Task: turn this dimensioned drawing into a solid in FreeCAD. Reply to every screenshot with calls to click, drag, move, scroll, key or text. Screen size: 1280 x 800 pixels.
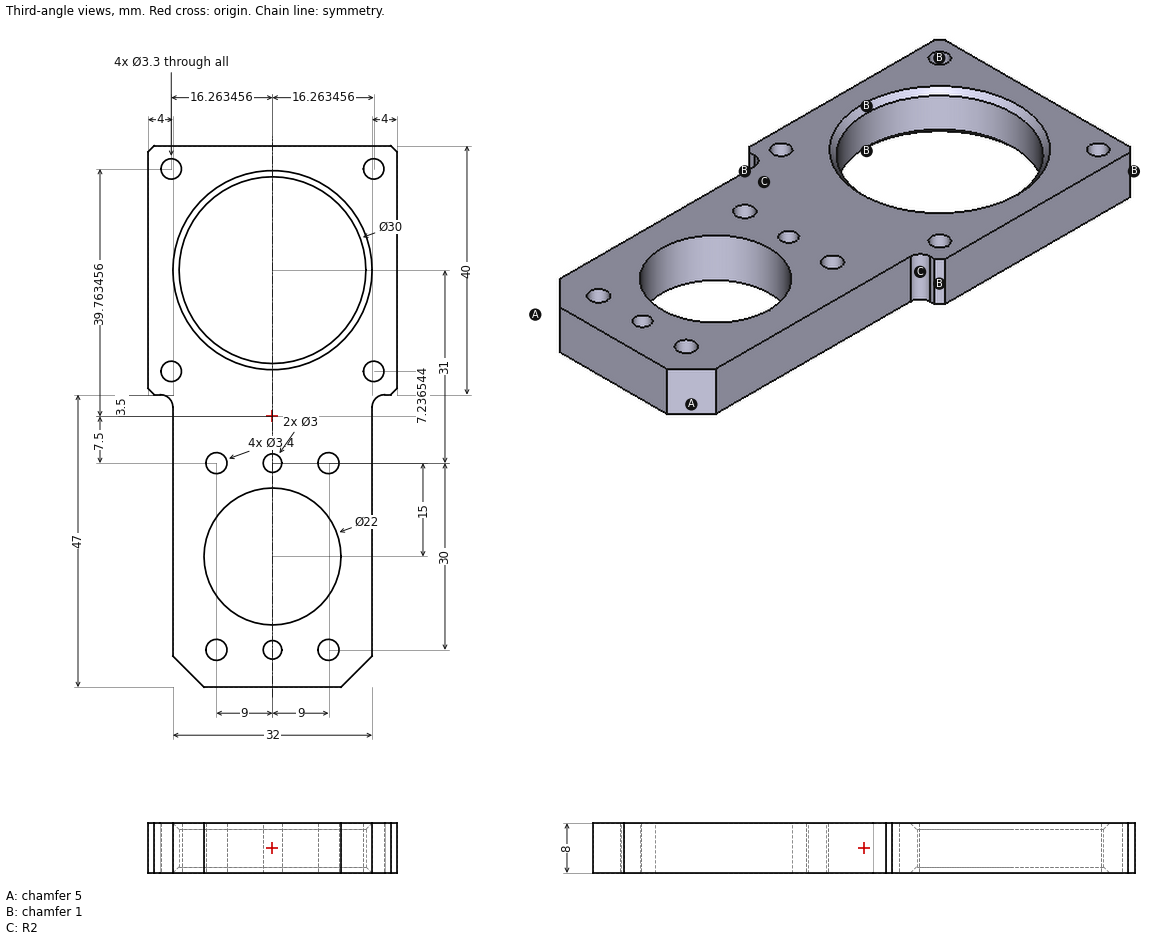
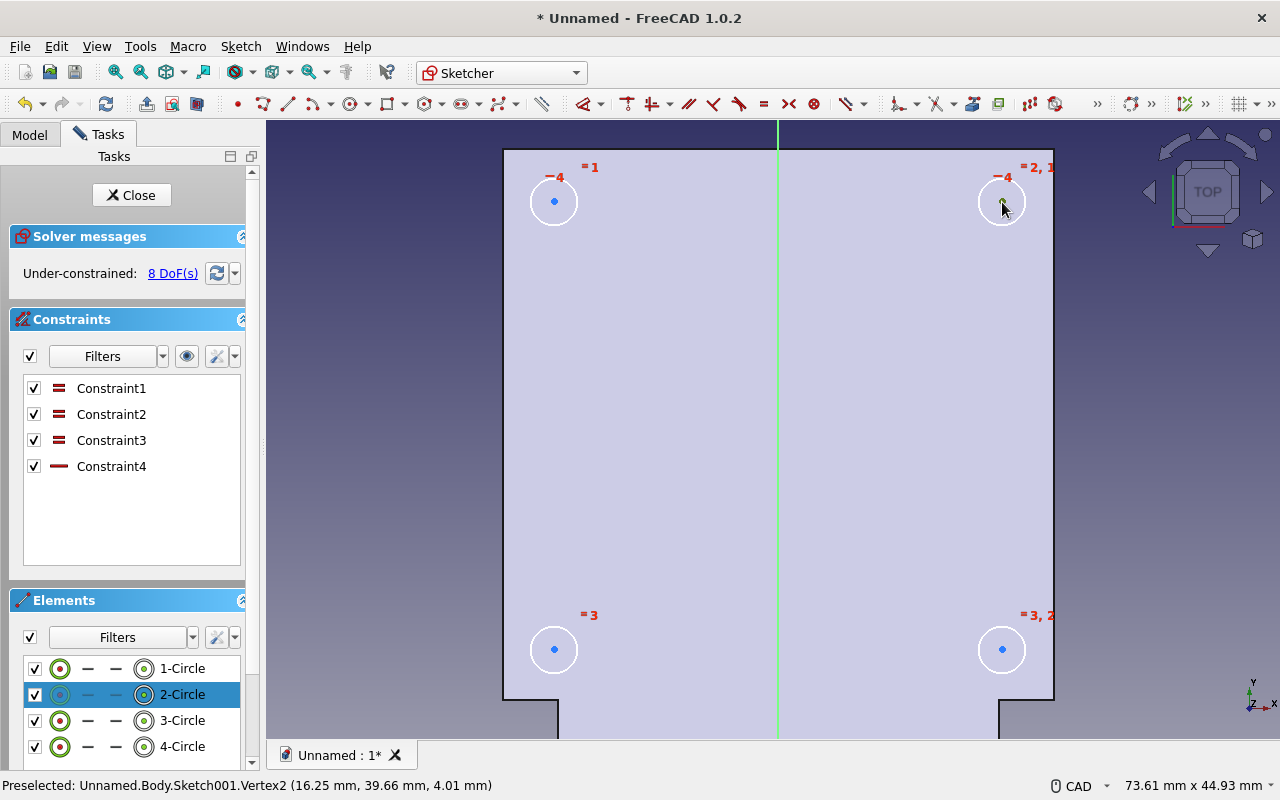
click(1002, 650)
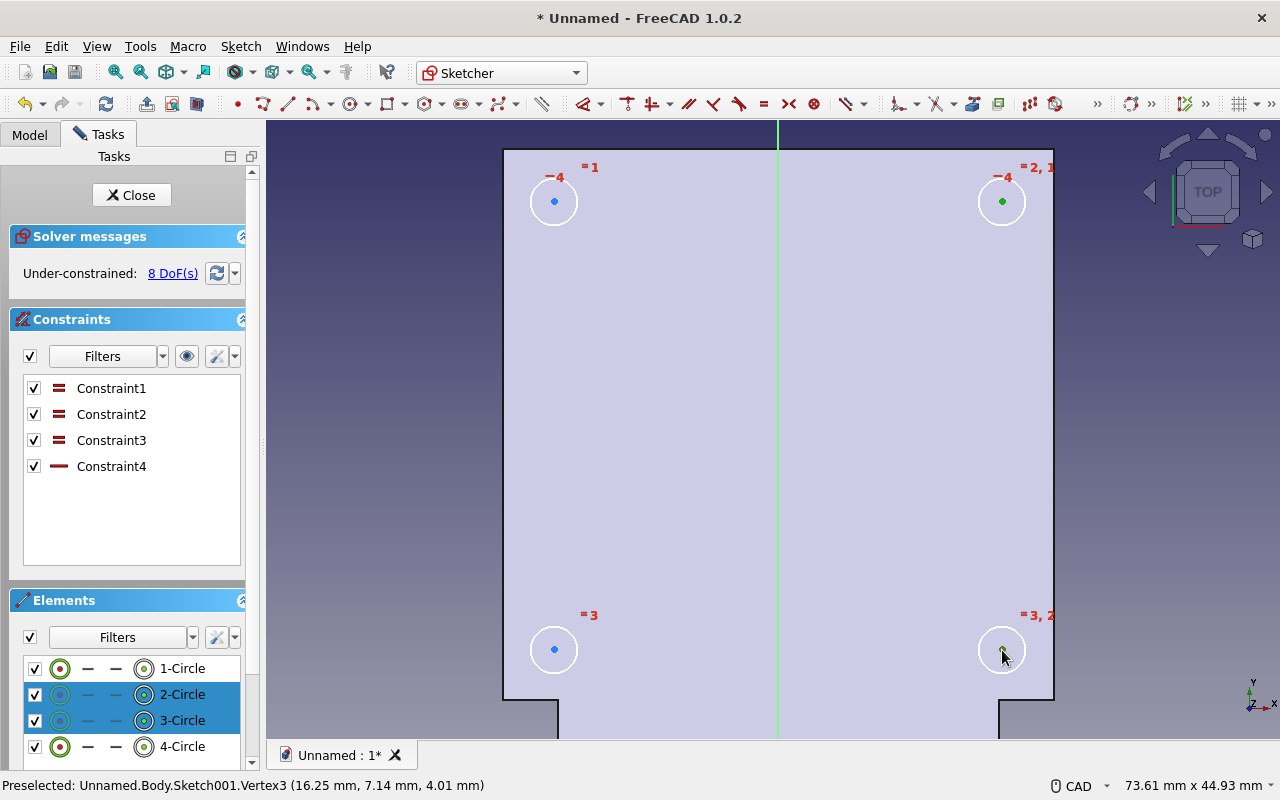
click(670, 104)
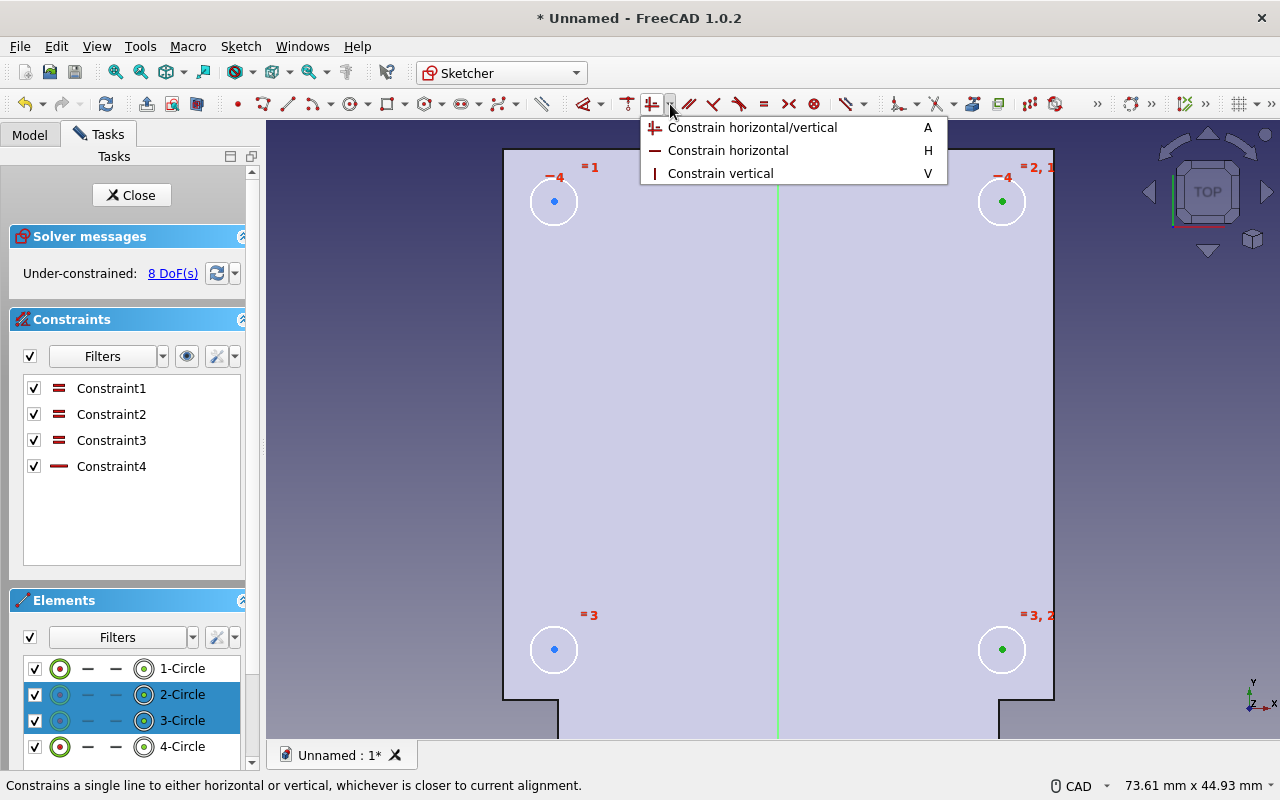
click(794, 174)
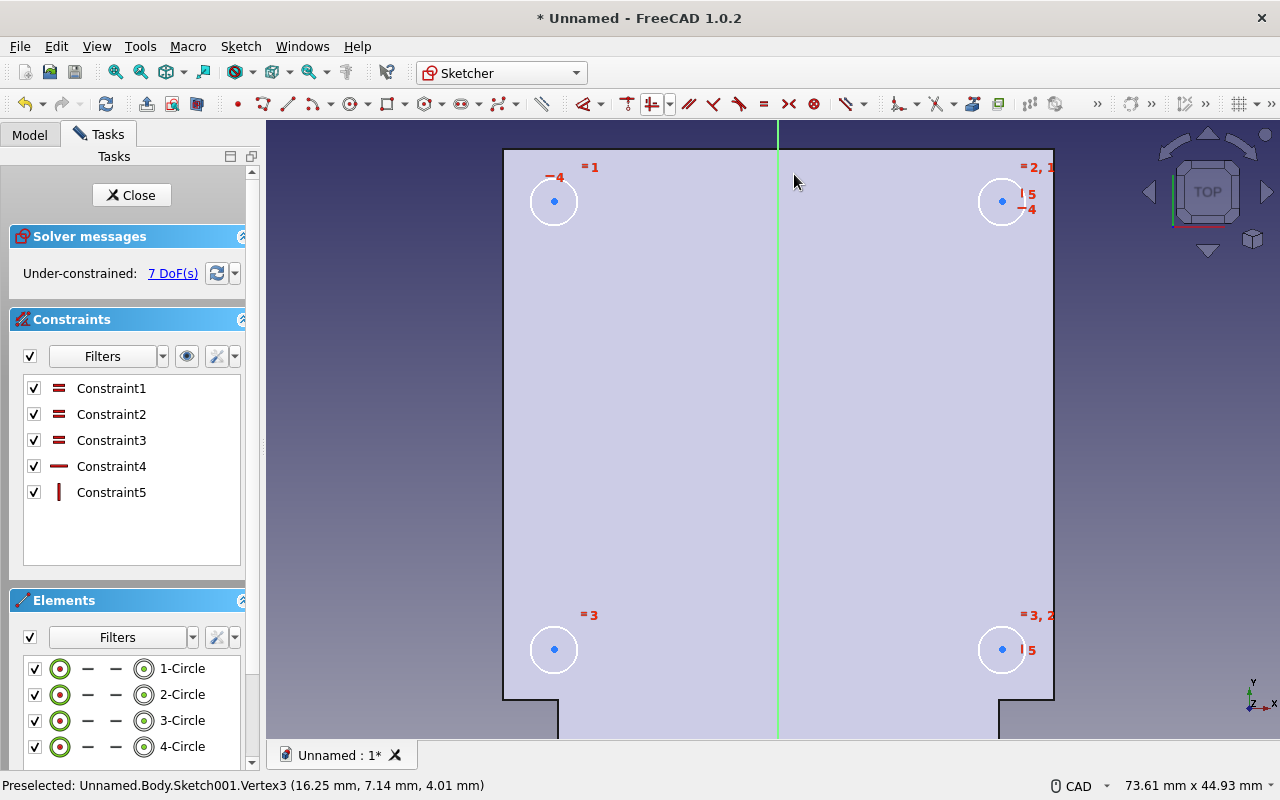
click(554, 202)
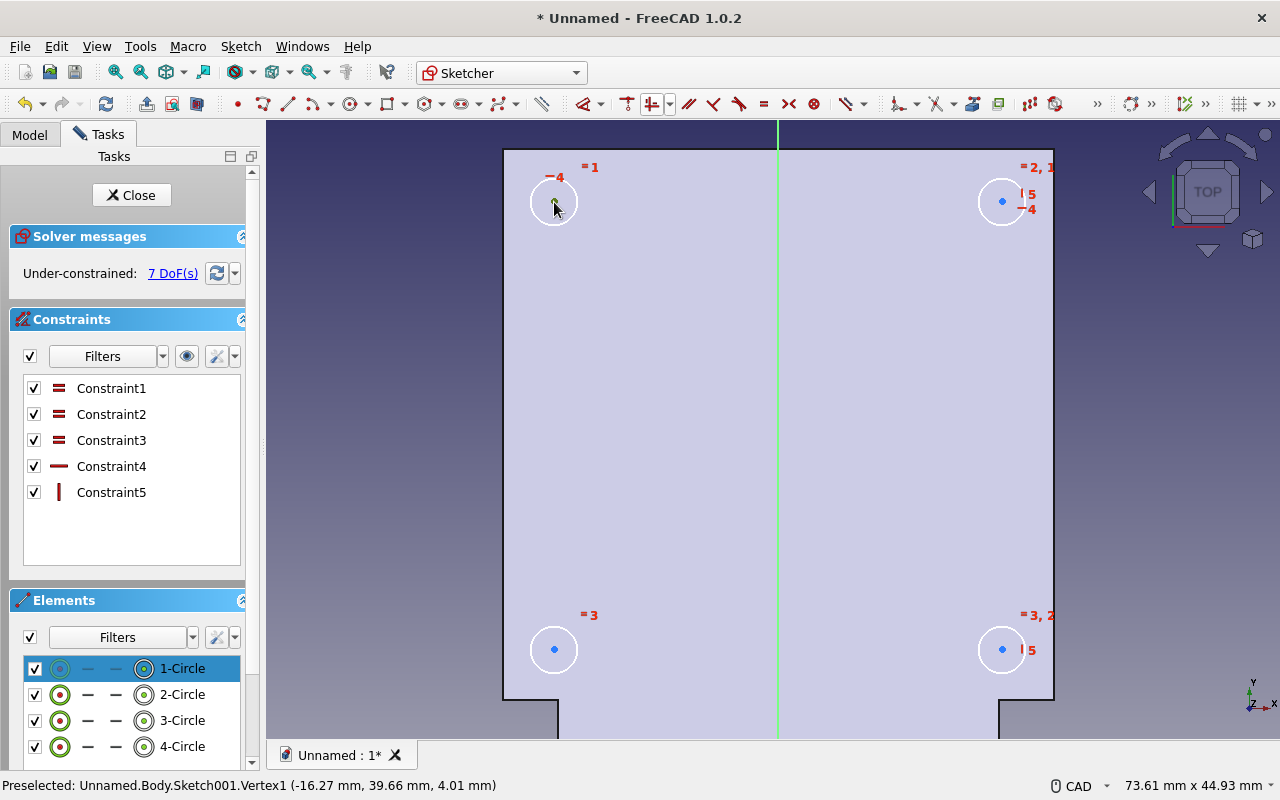
click(554, 650)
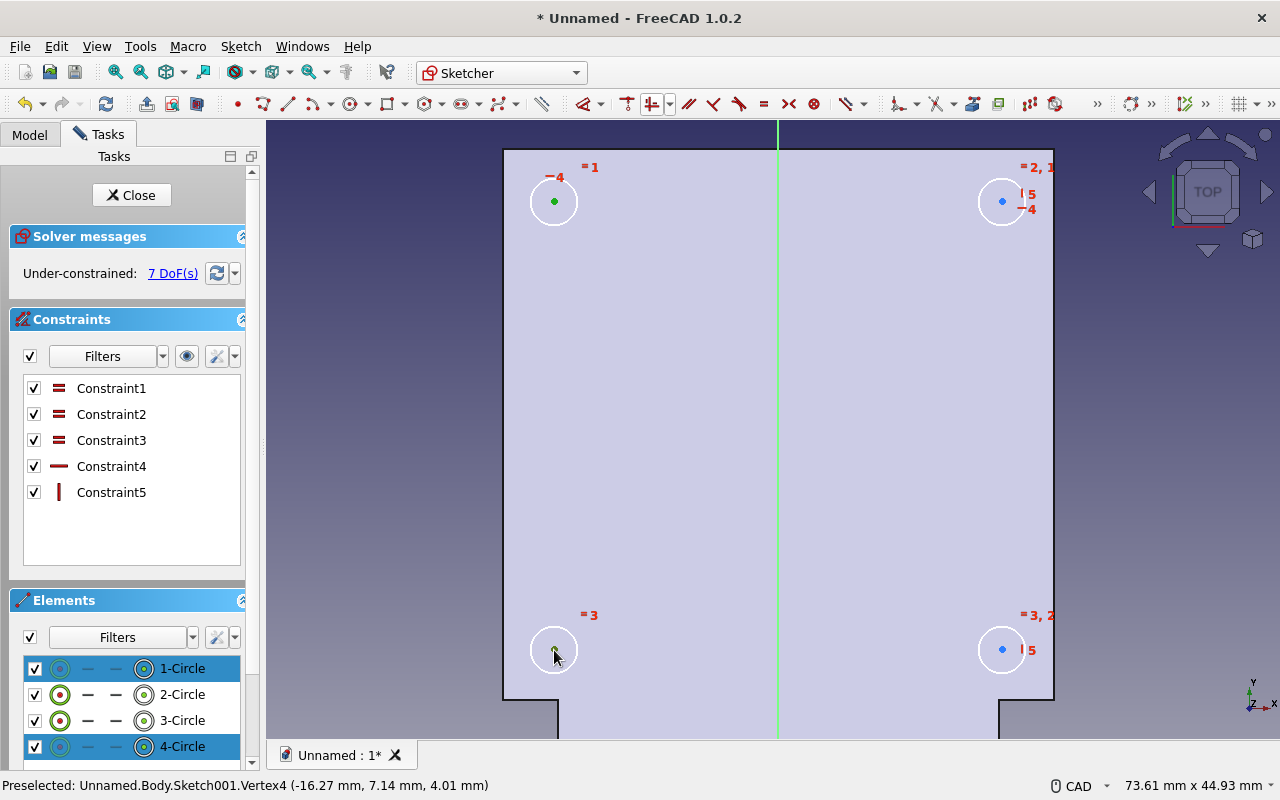
click(670, 104)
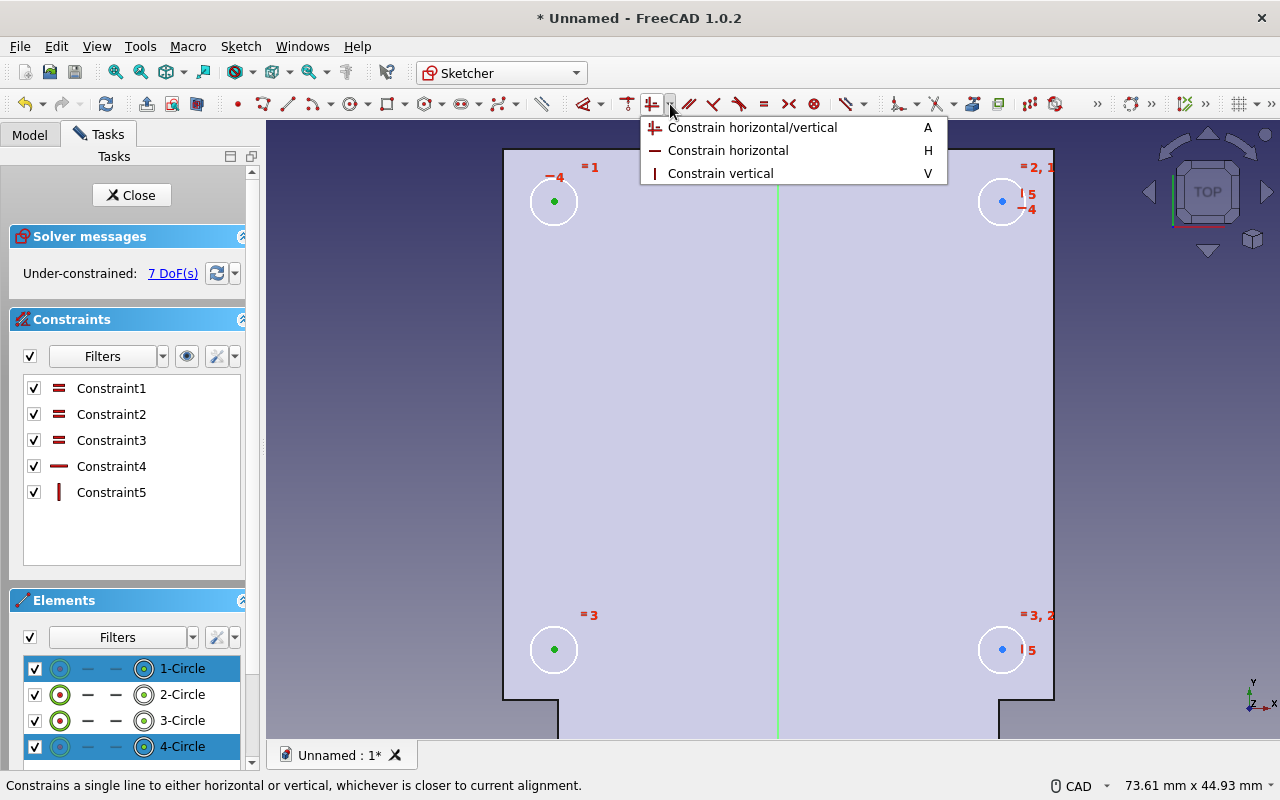
click(794, 174)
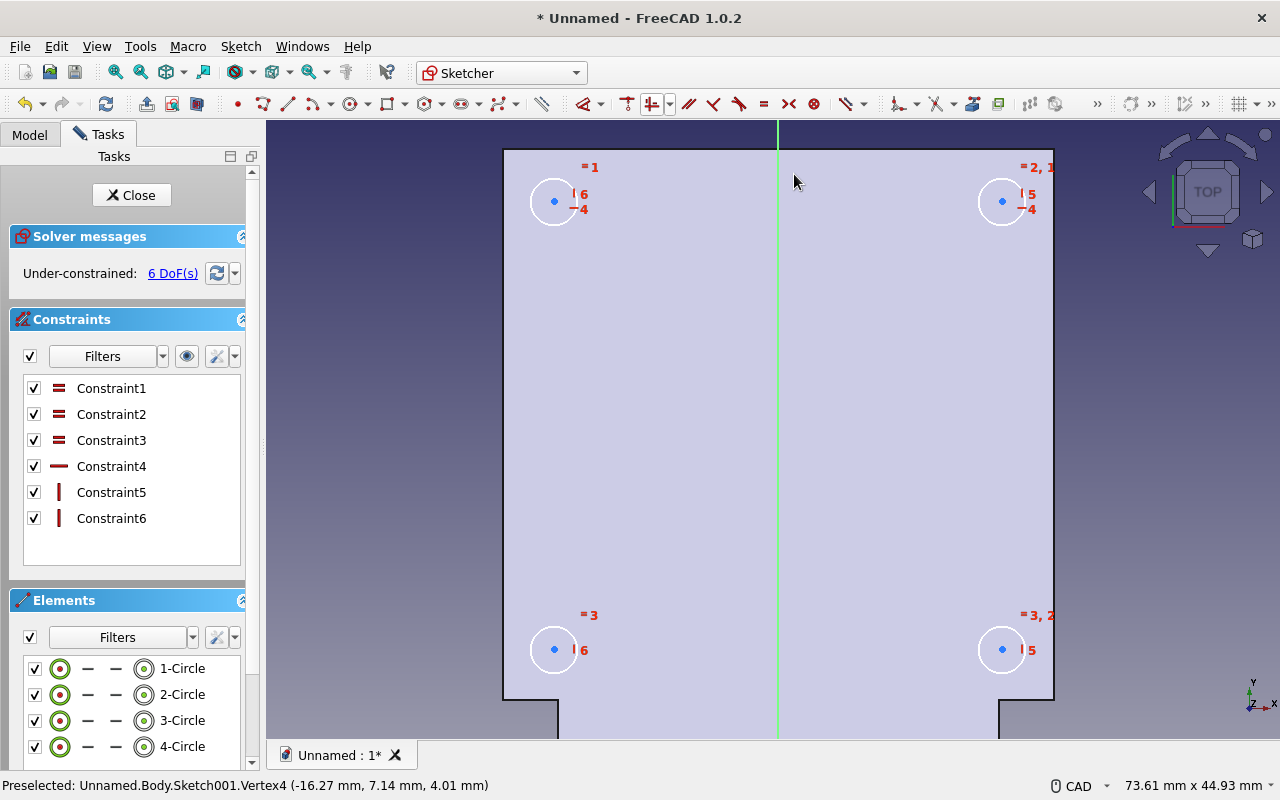
click(1002, 650)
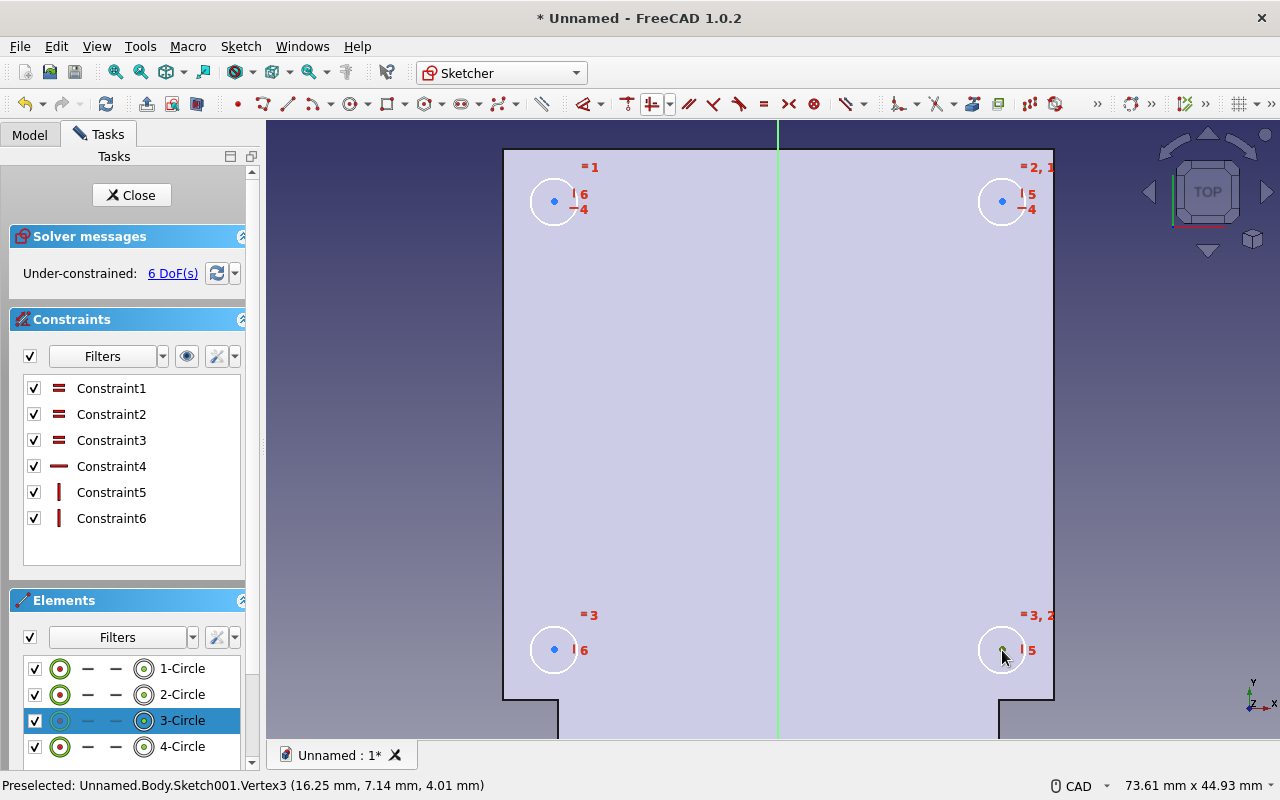
click(554, 650)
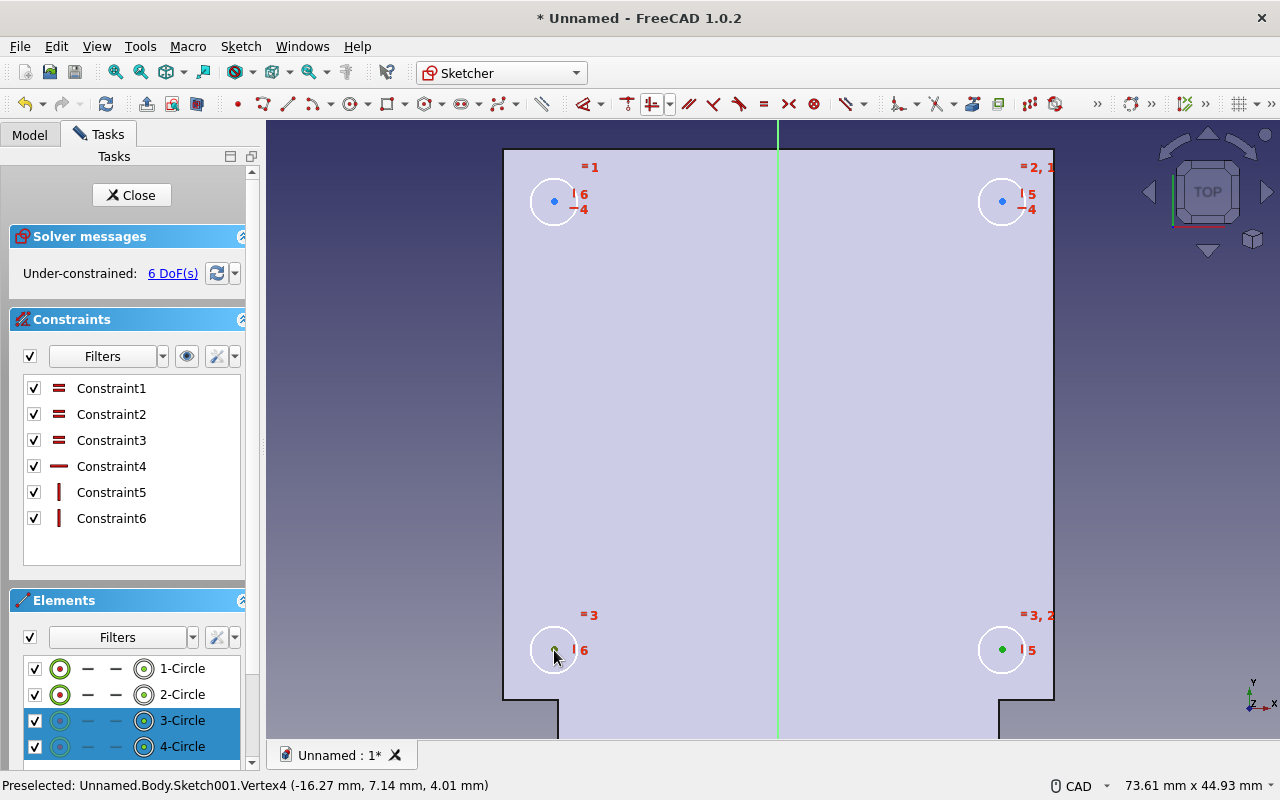
key(h)